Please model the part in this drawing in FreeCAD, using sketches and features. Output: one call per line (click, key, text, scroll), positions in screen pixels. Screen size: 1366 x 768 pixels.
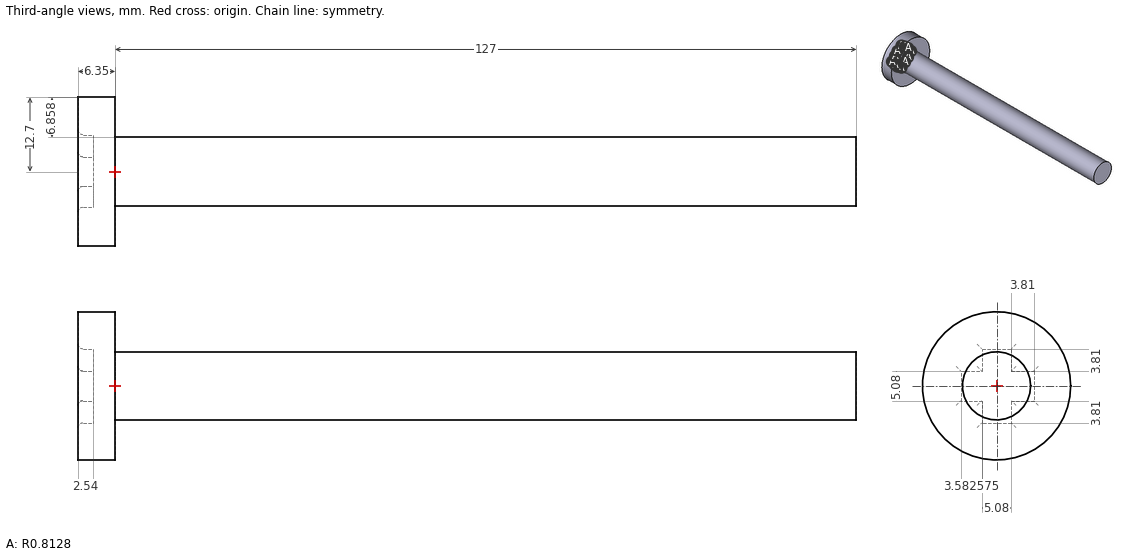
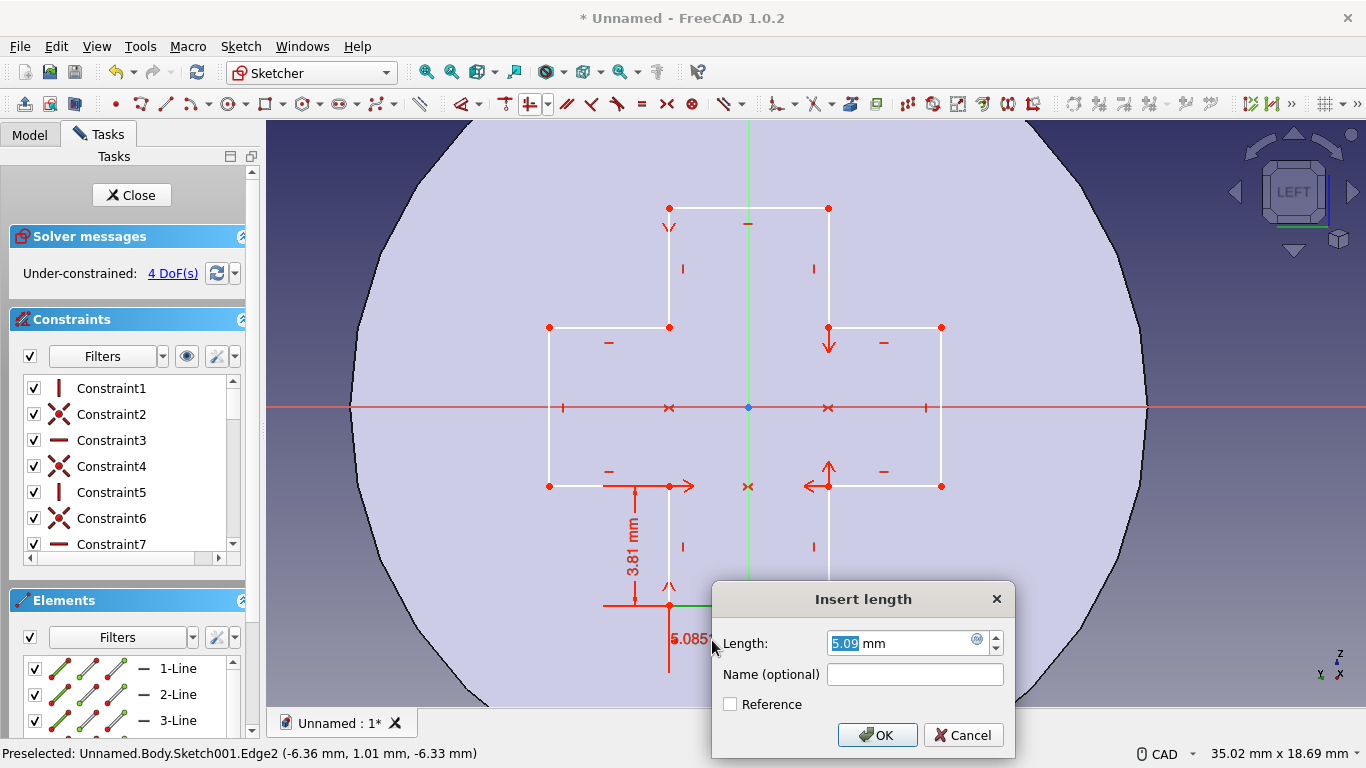
text(5.08)
key(Return)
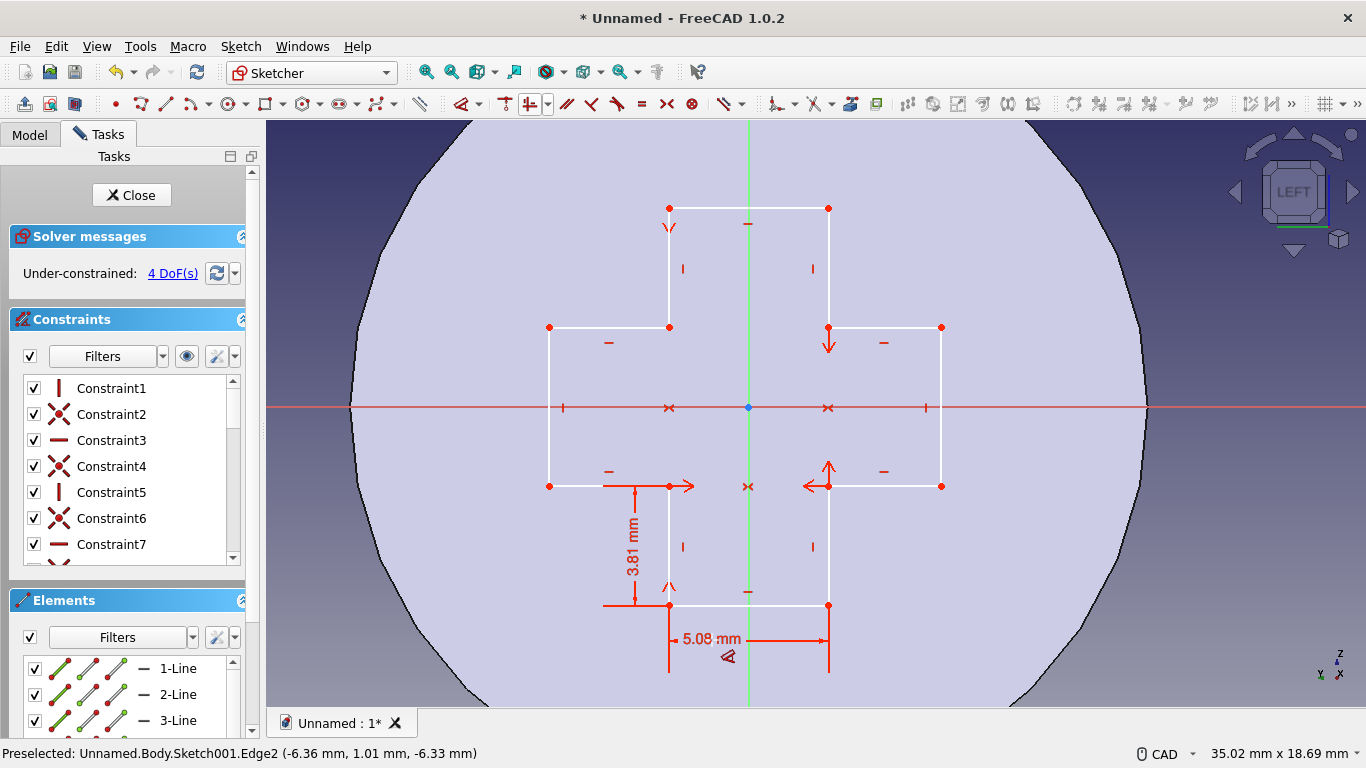
click(941, 439)
click(975, 371)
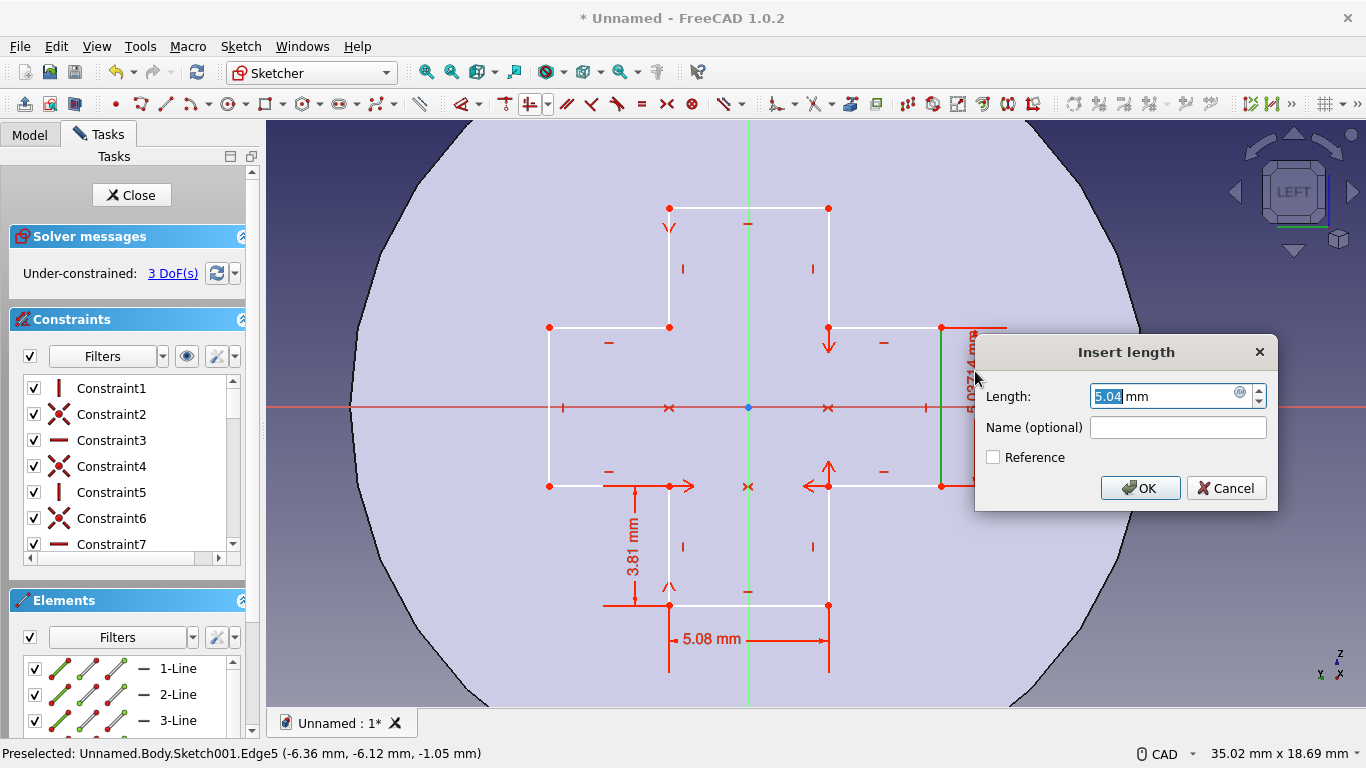
text(5.08)
key(Return)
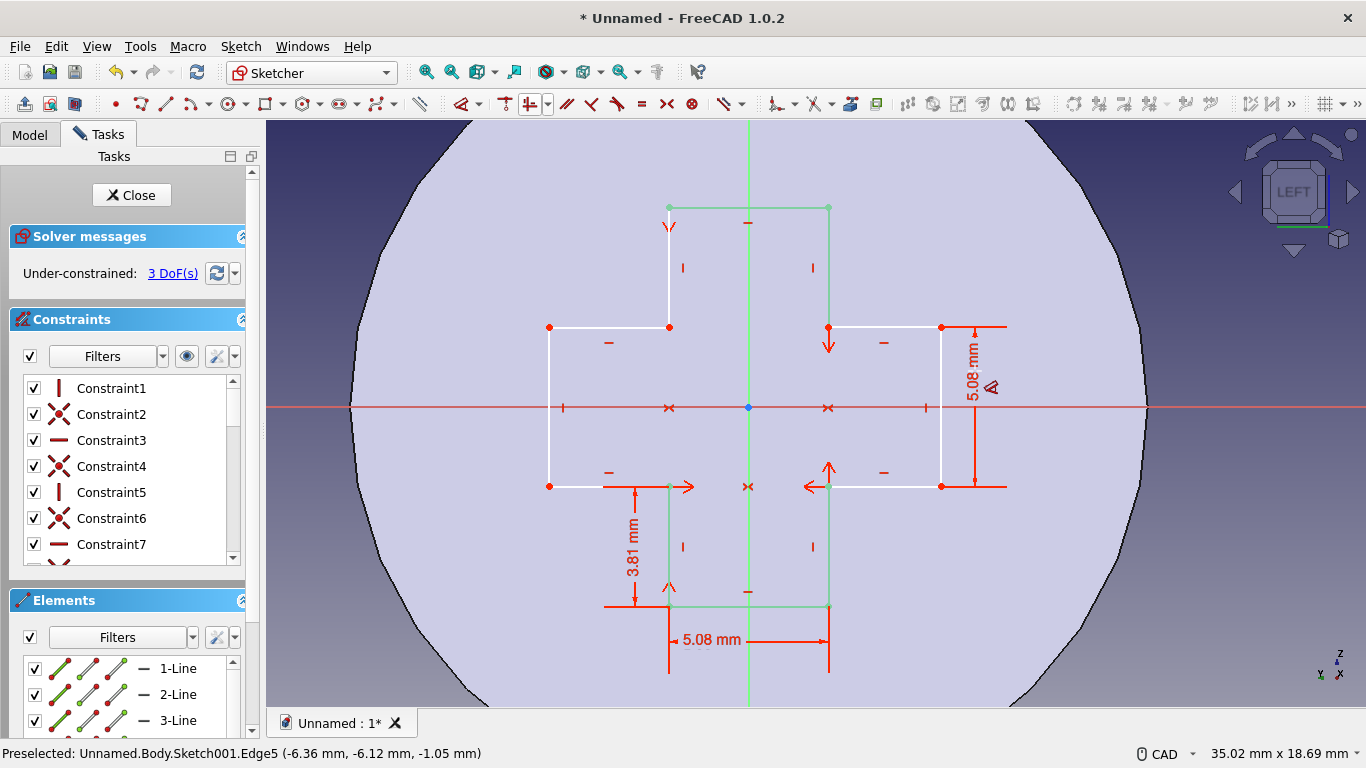
click(669, 244)
click(635, 268)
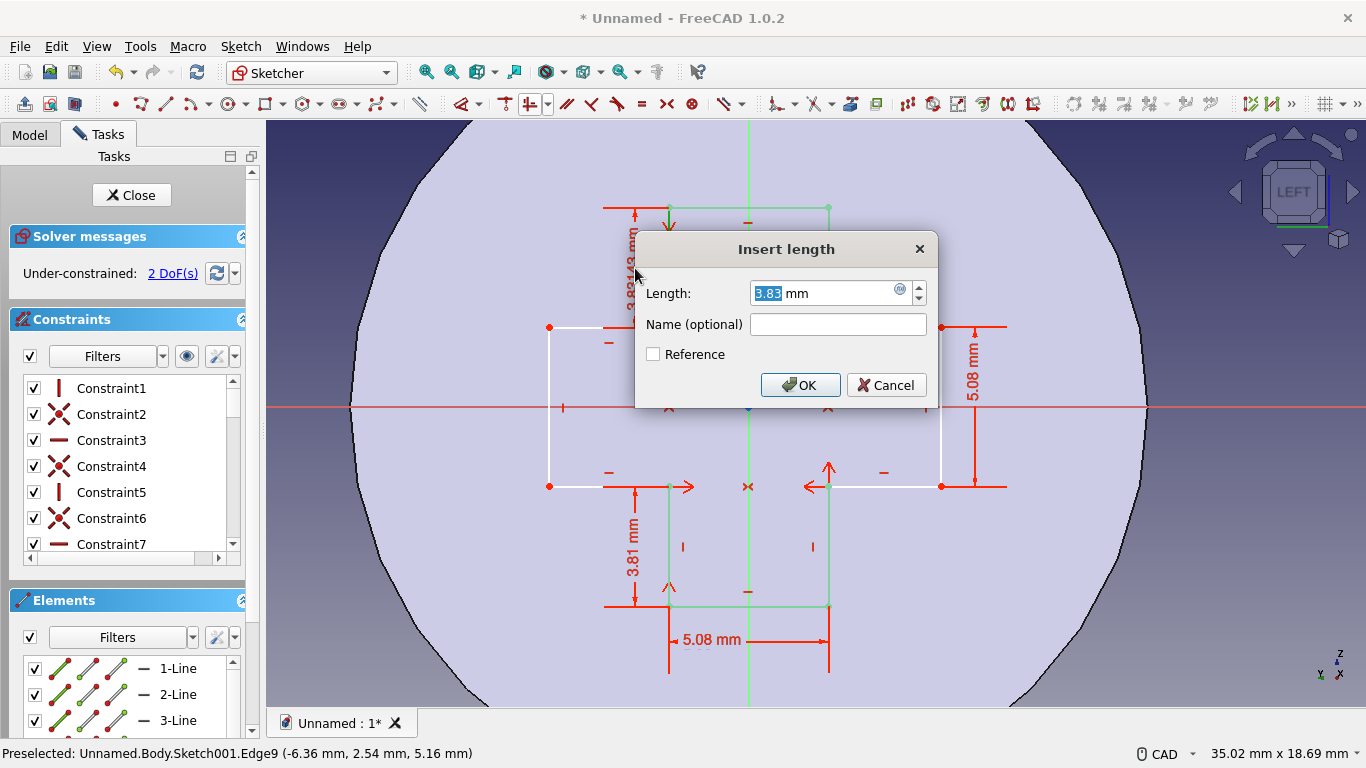
text(3.81)
key(Return)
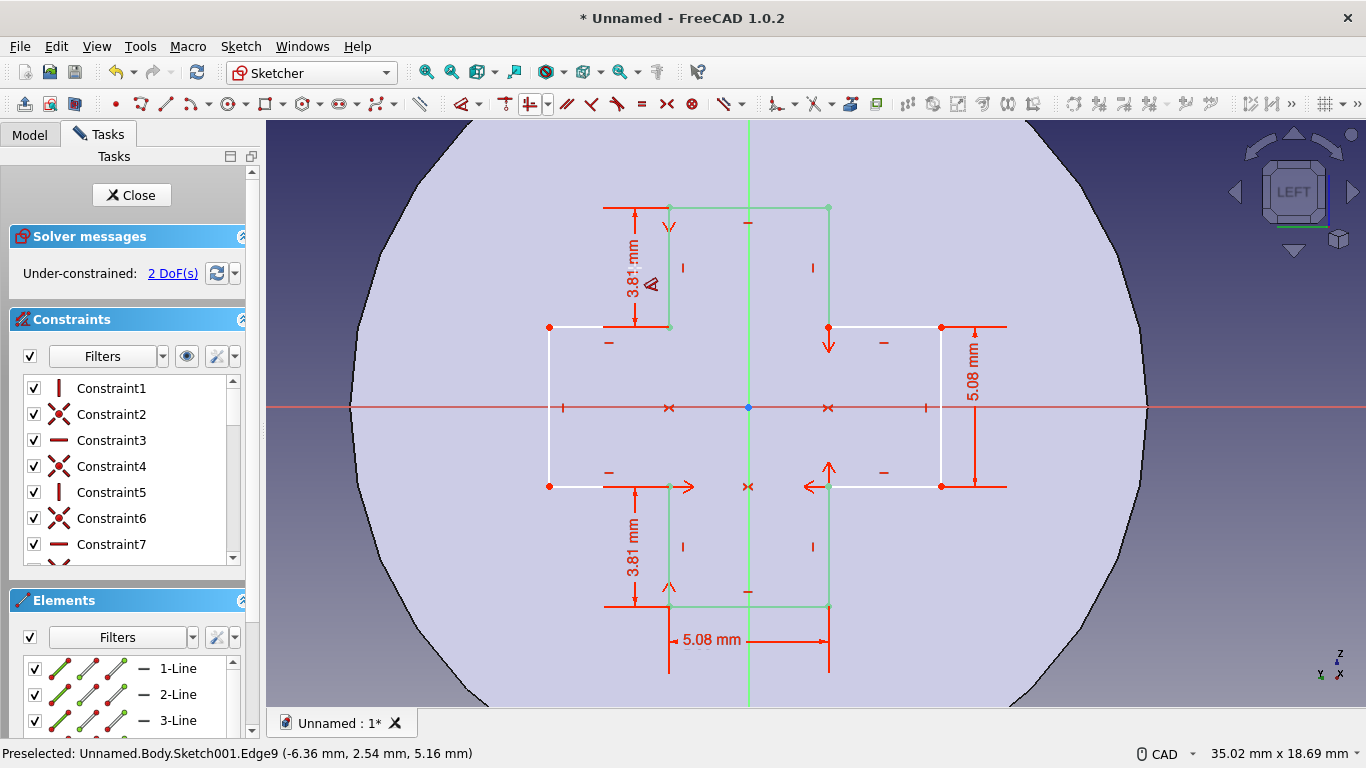
click(633, 327)
click(609, 293)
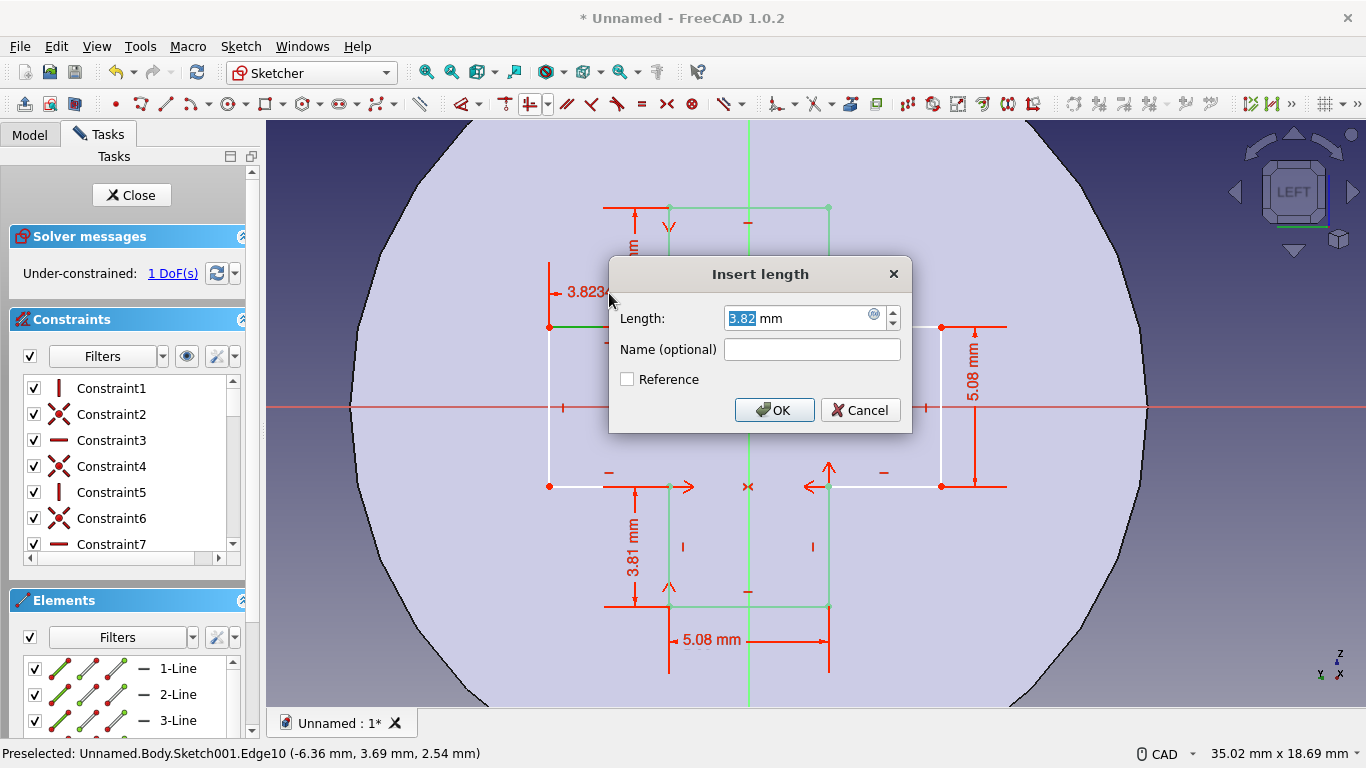
text(3.81)
key(Return)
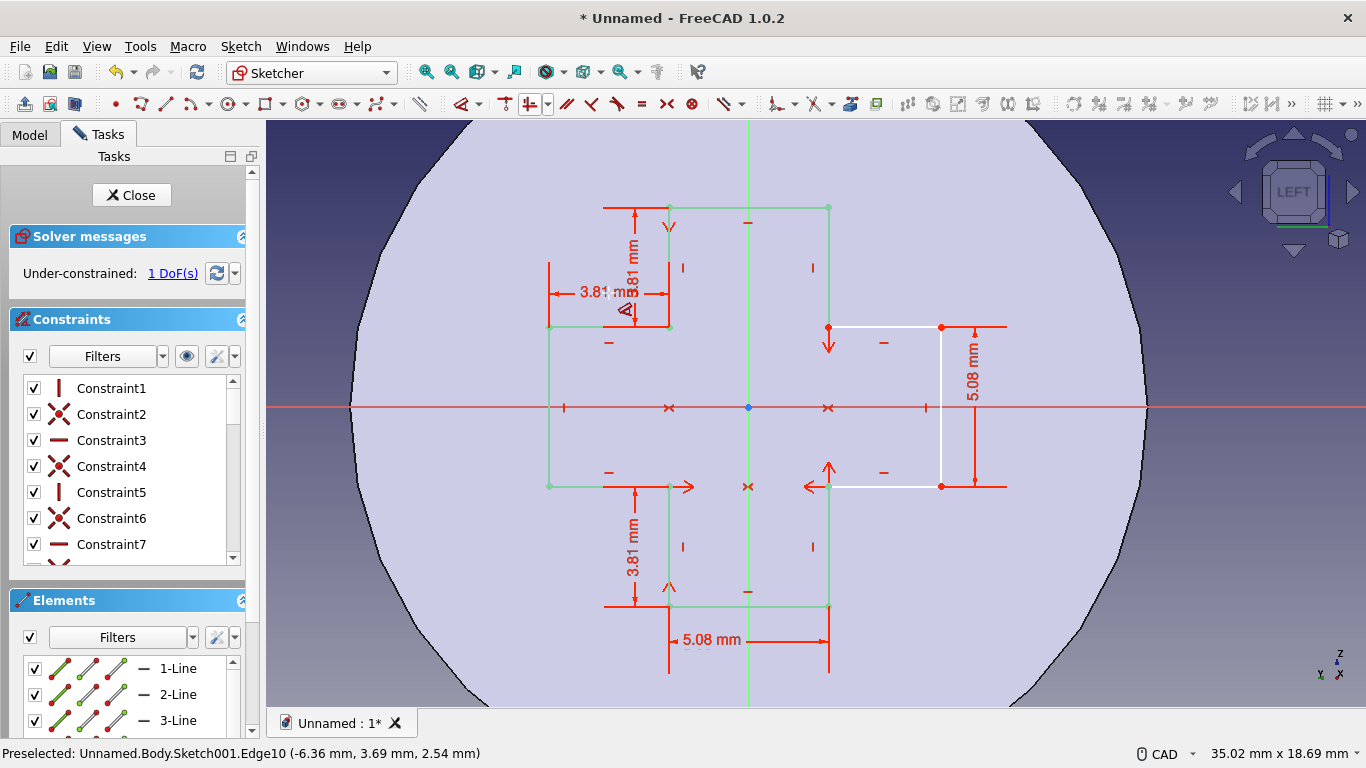
click(862, 487)
click(885, 521)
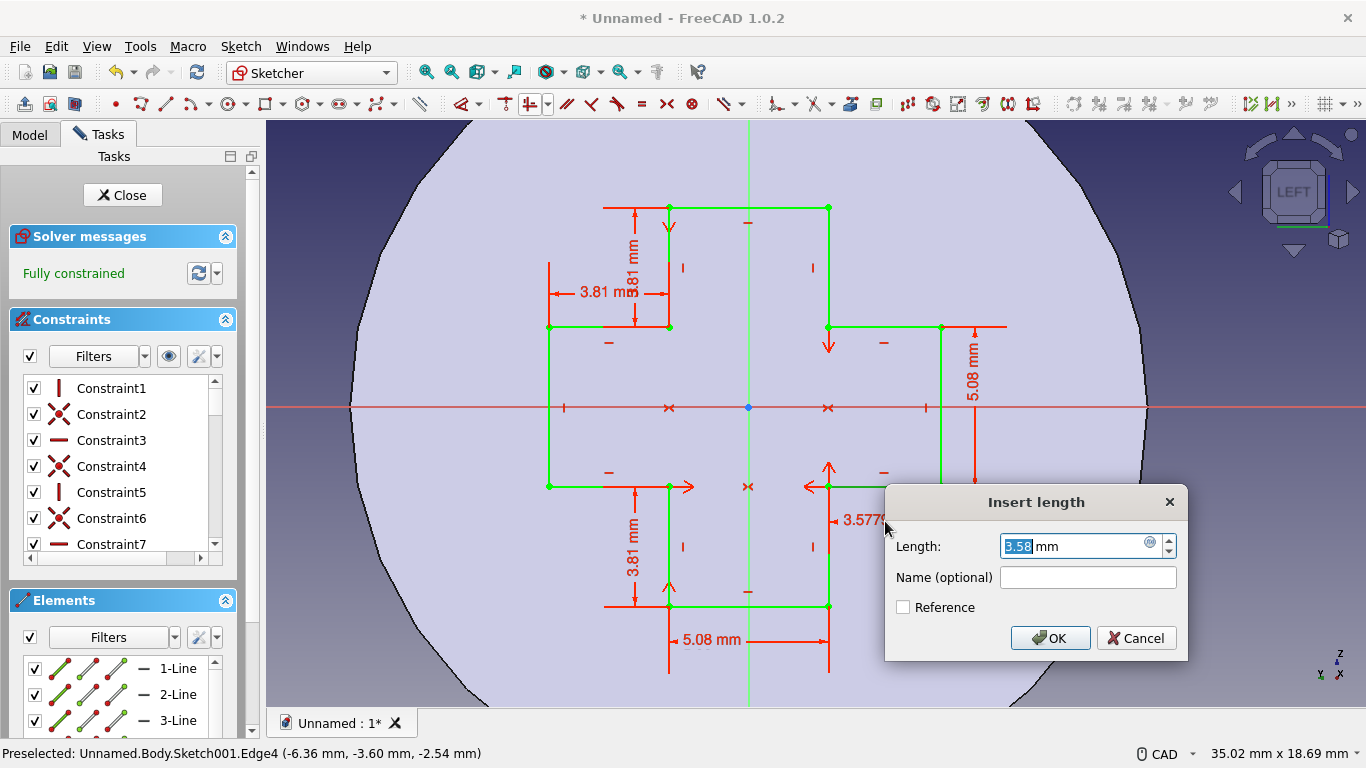
text(3.582575)
key(Return)
key(Escape)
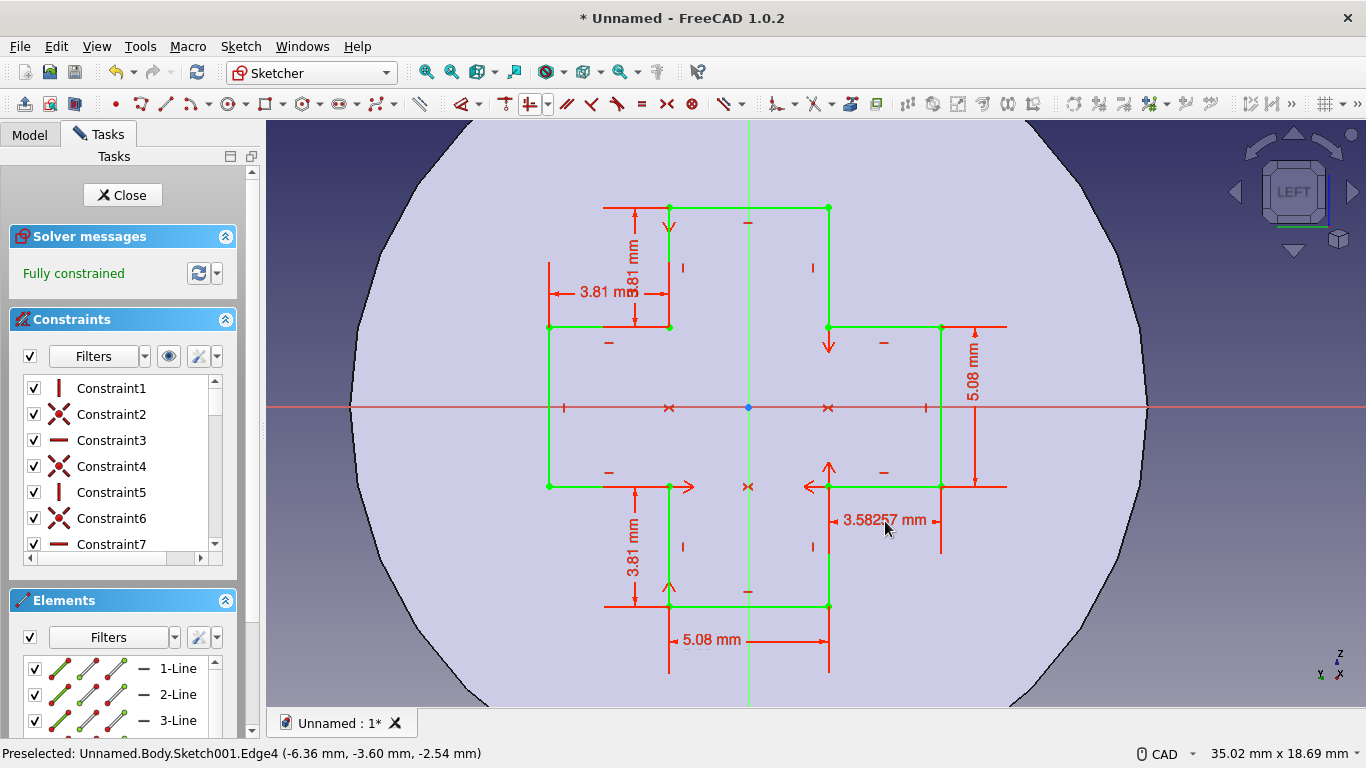
click(123, 195)